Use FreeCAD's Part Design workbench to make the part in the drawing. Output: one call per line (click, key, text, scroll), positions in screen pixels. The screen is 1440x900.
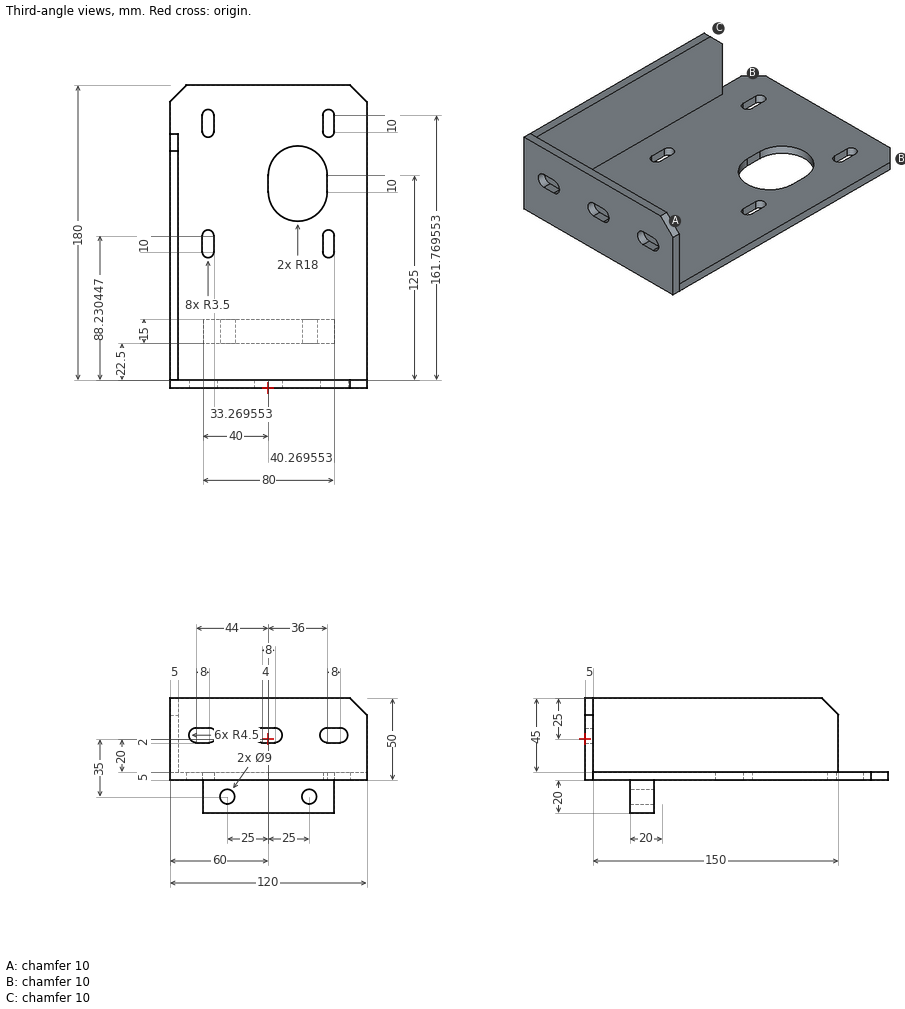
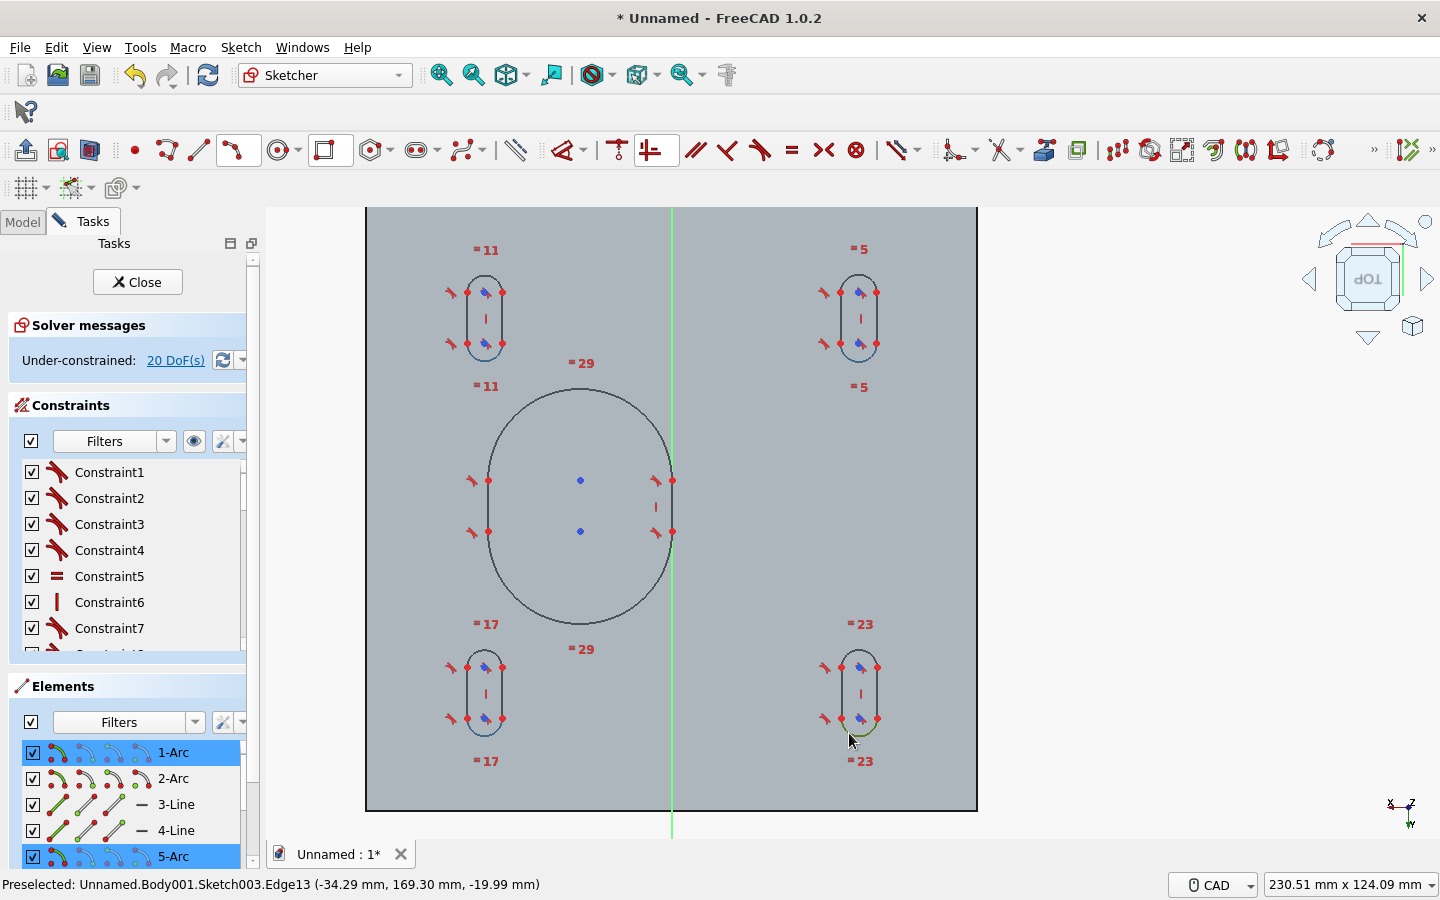
key(e)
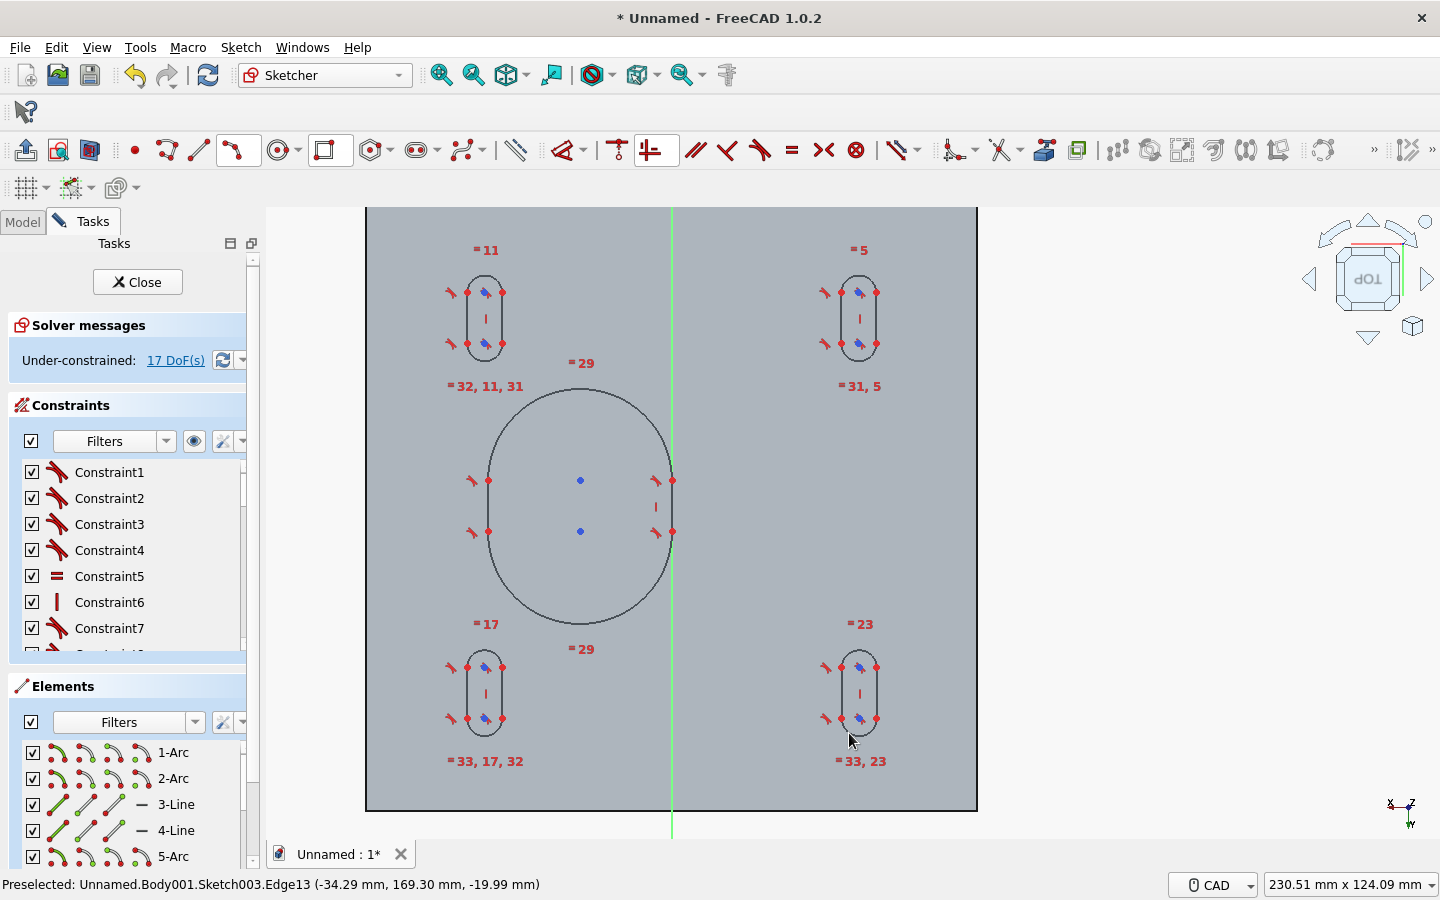
key(d)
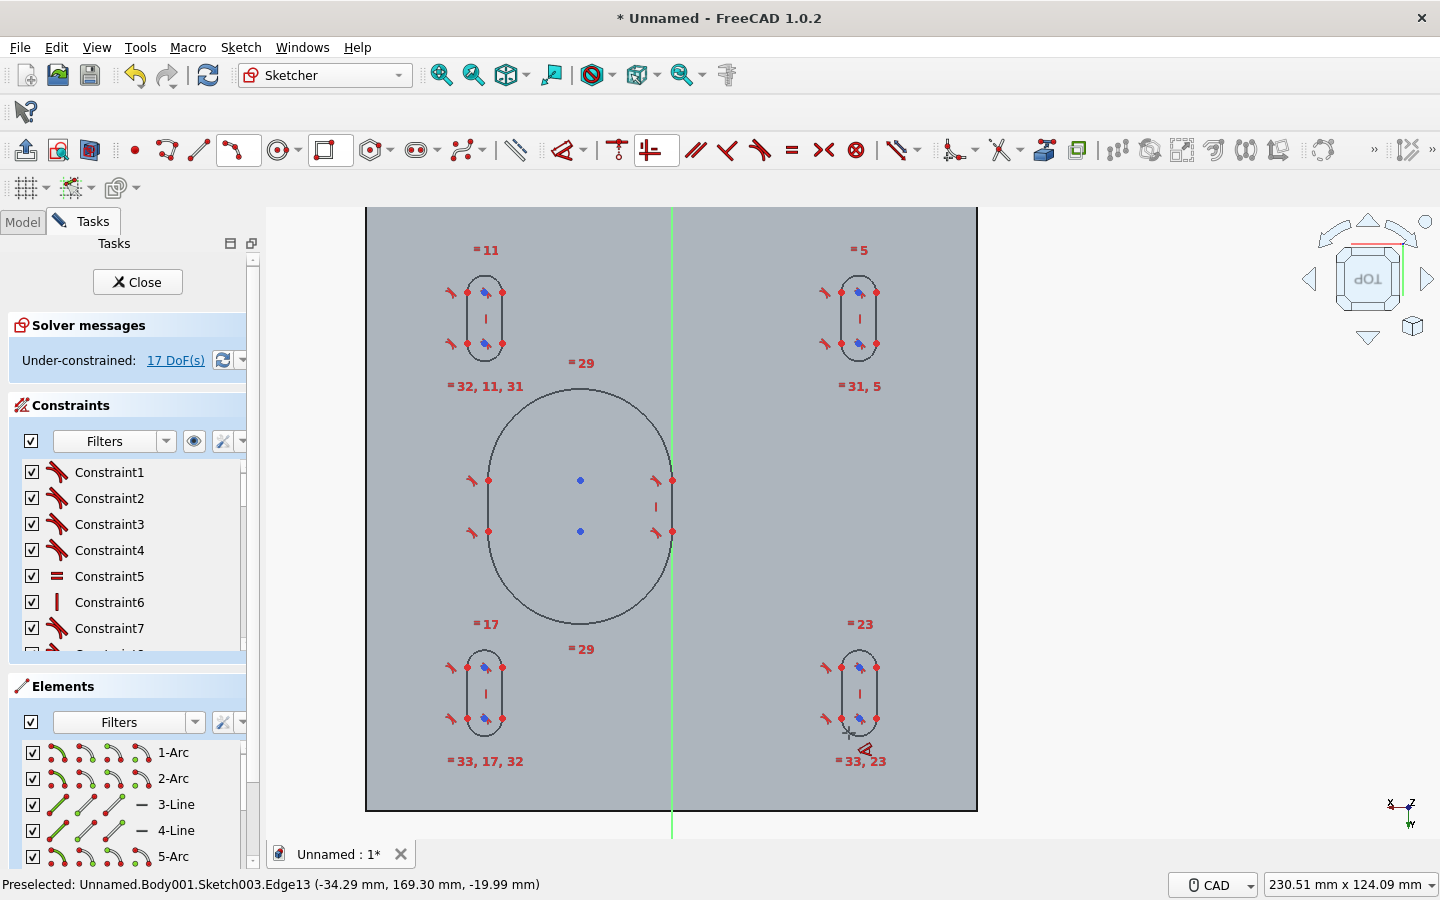
scroll(848, 358, up, 5)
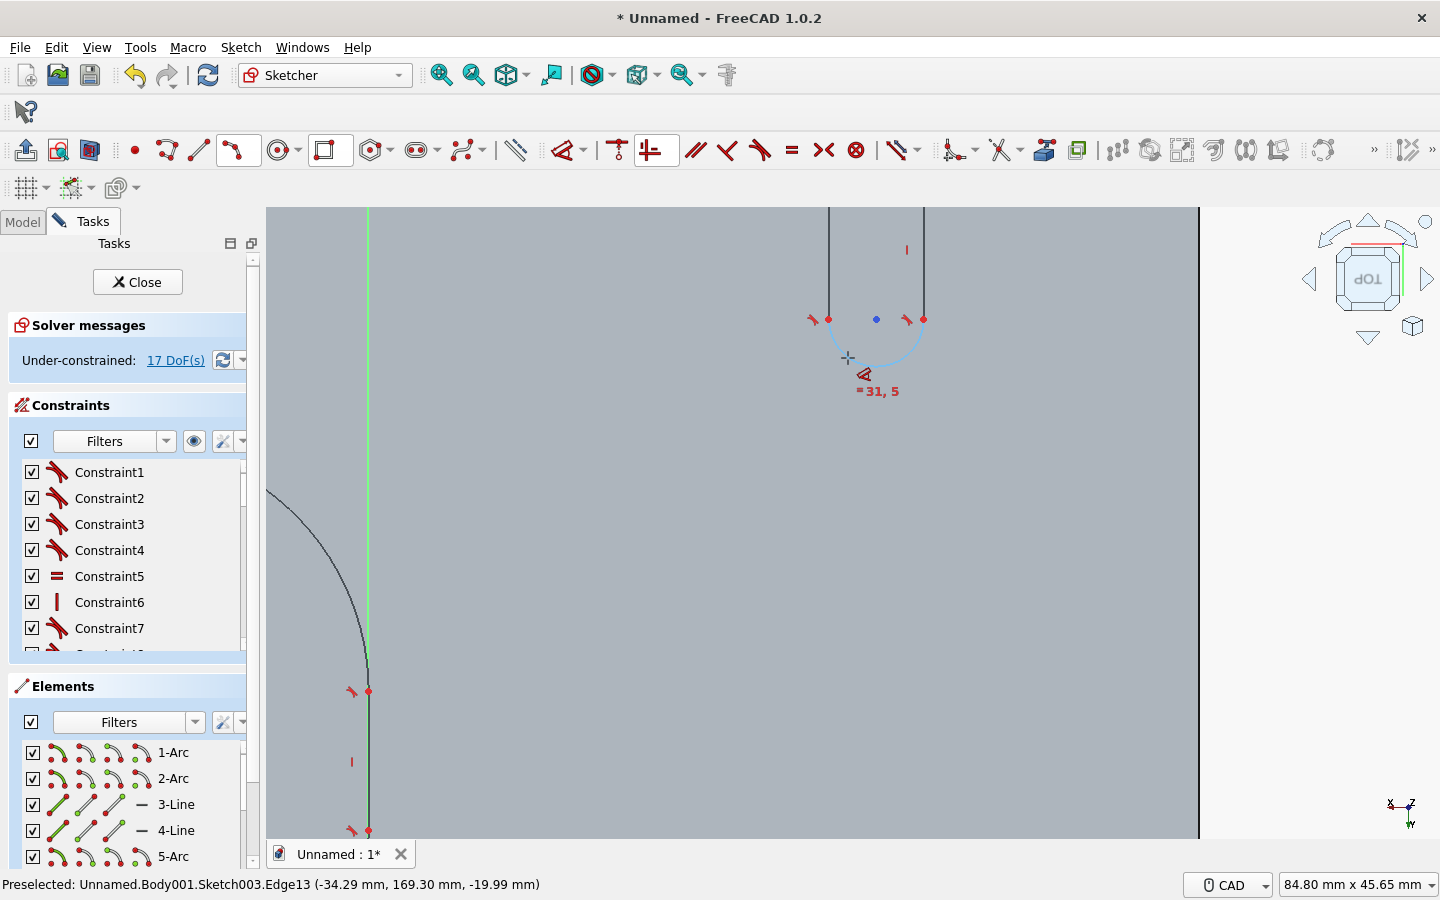
click(849, 358)
click(831, 384)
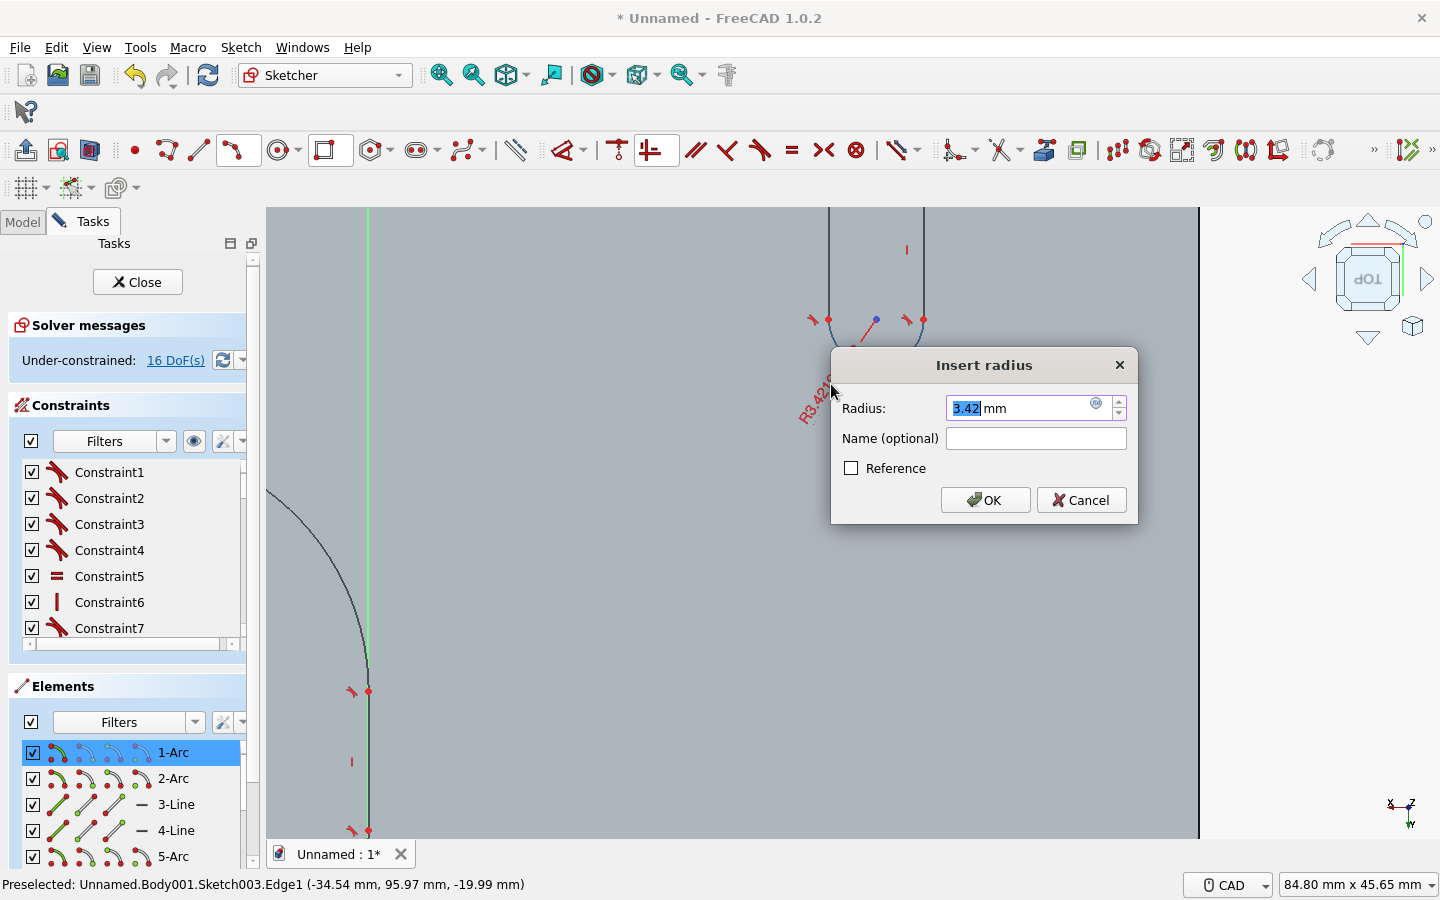
text(3.5)
key(Return)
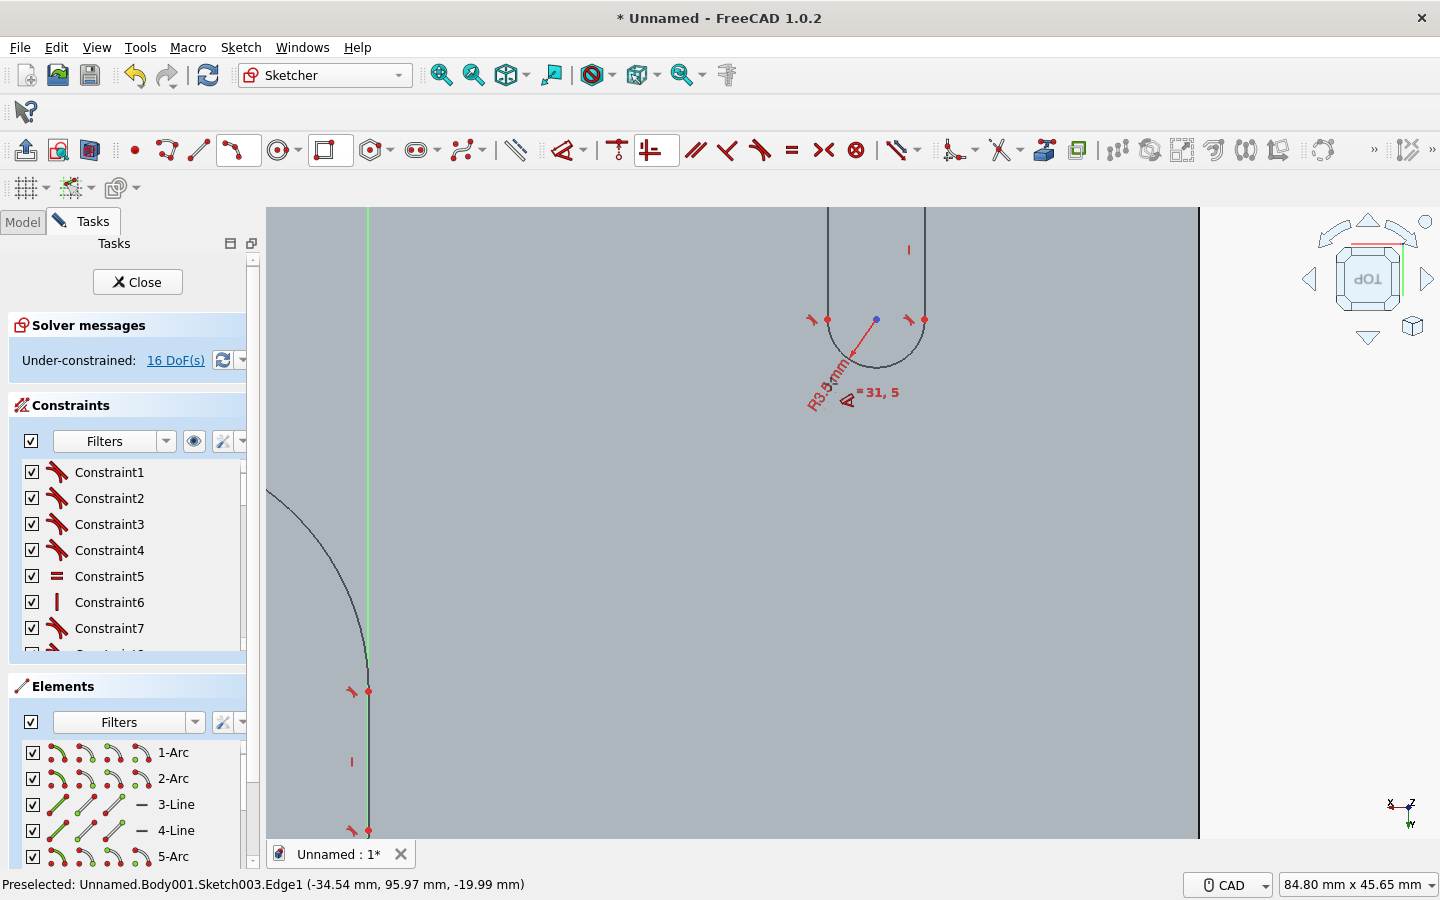
scroll(867, 579, down, 9)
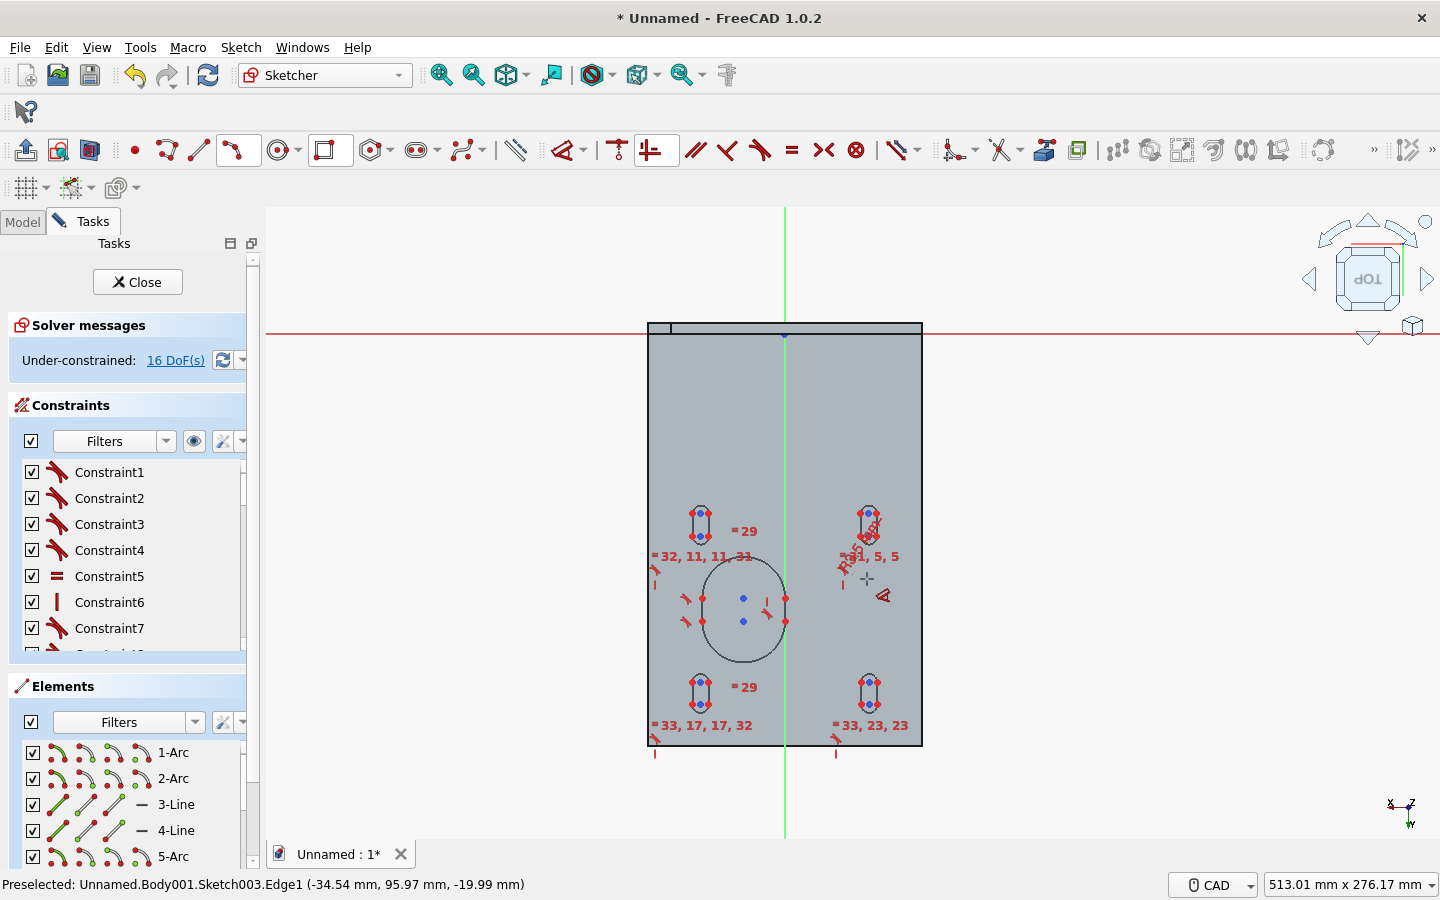
click(719, 655)
click(677, 653)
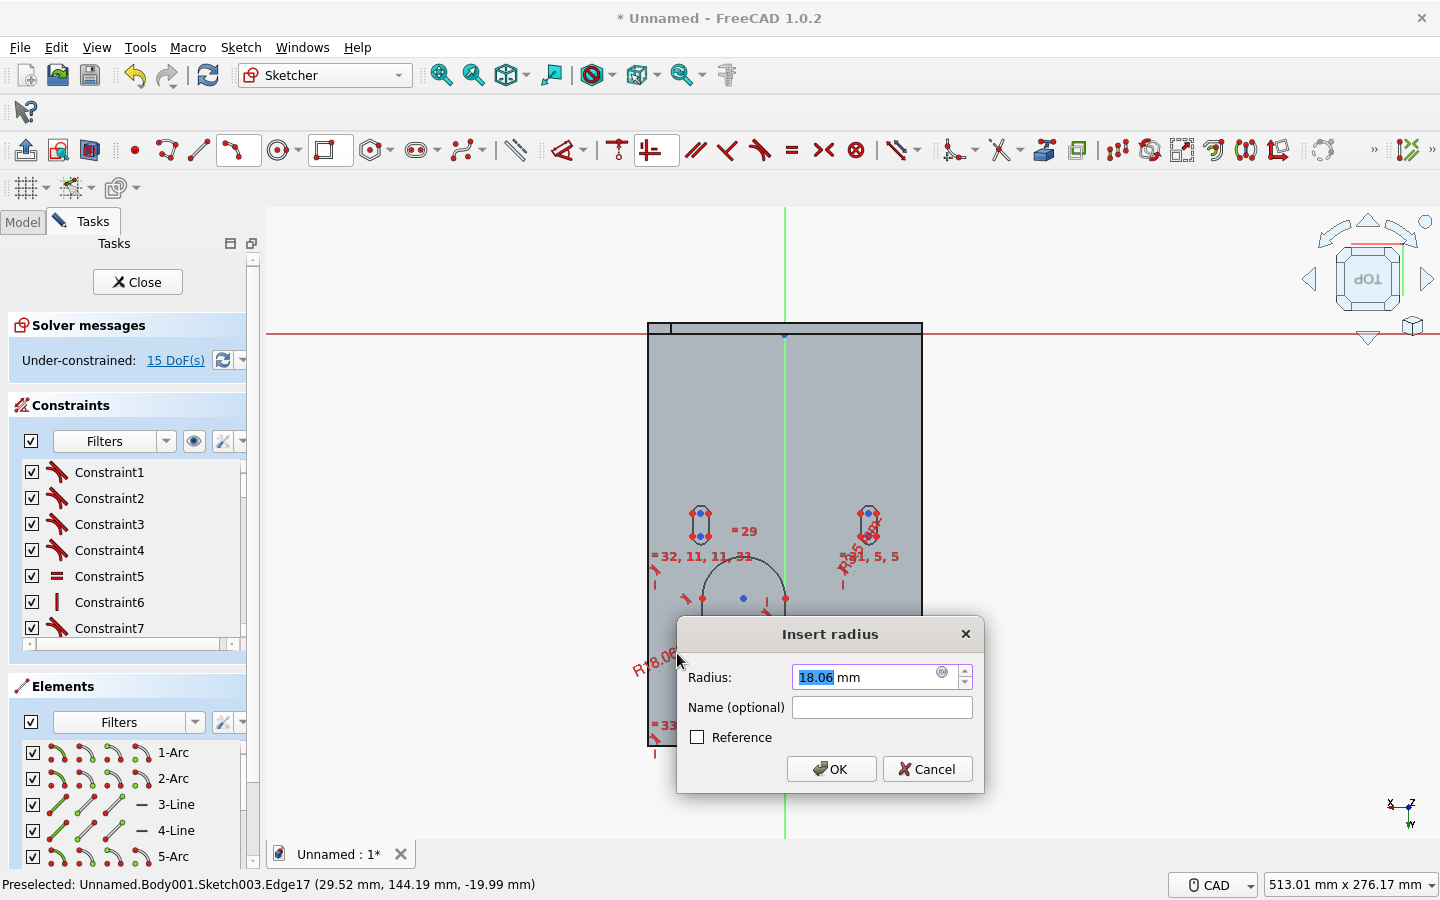
text(18)
key(Return)
key(Escape)